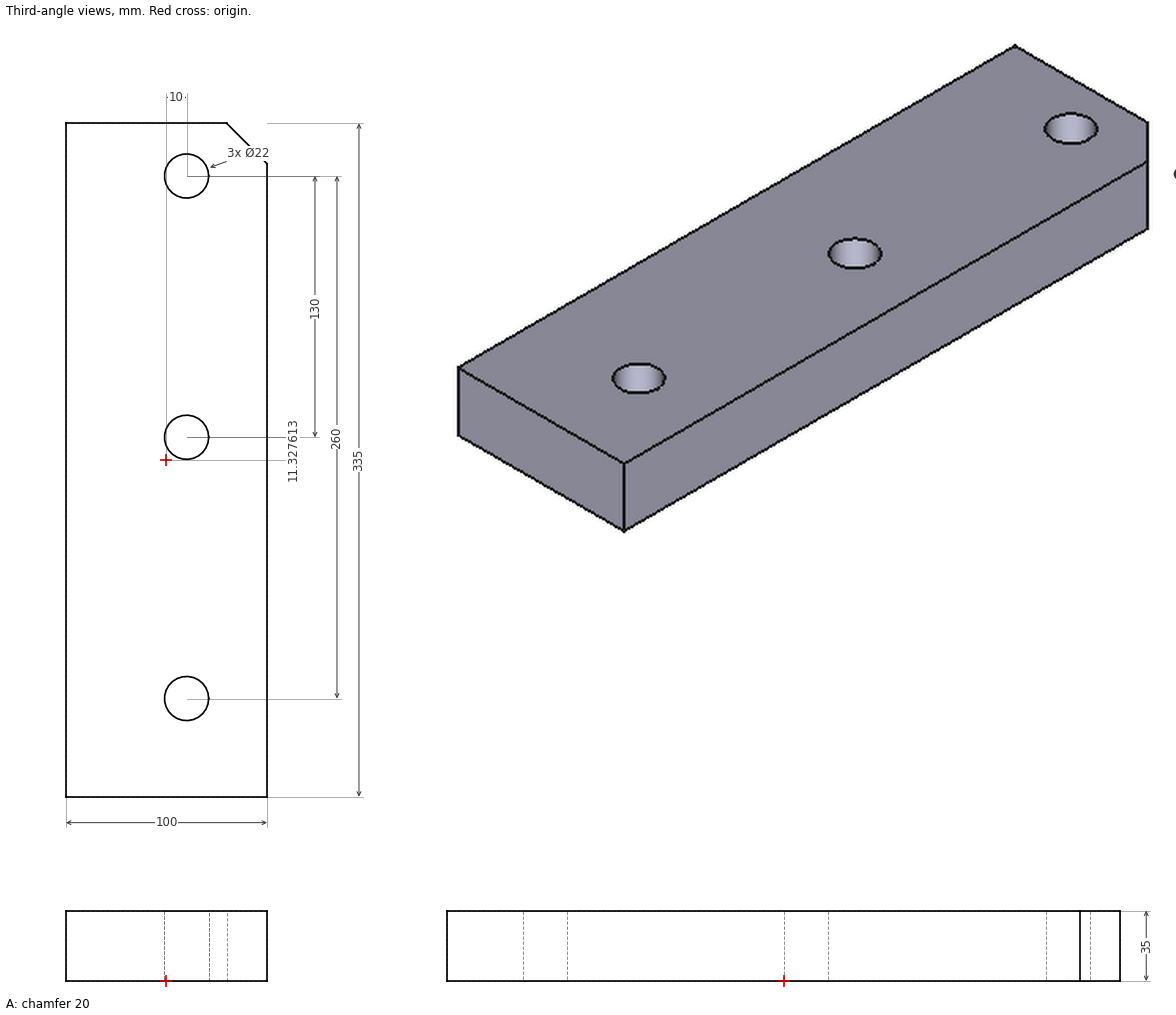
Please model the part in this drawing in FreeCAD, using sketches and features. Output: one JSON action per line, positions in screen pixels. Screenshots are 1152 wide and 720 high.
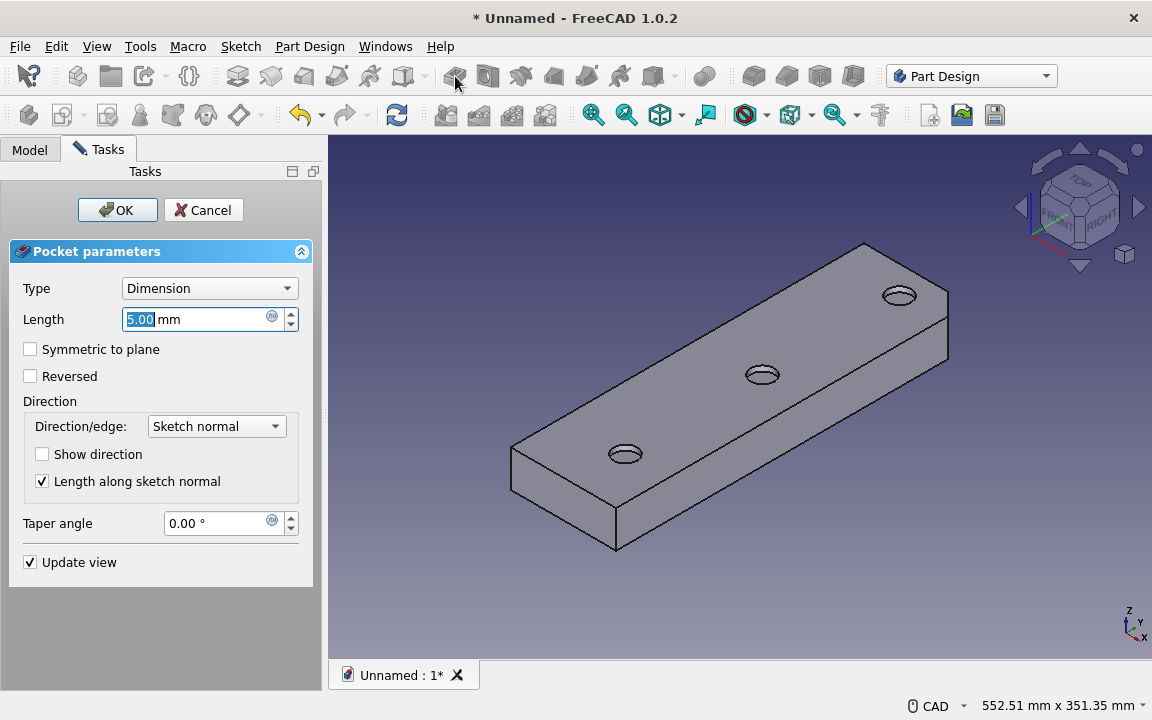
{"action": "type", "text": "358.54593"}
{"action": "key", "text": "Tab"}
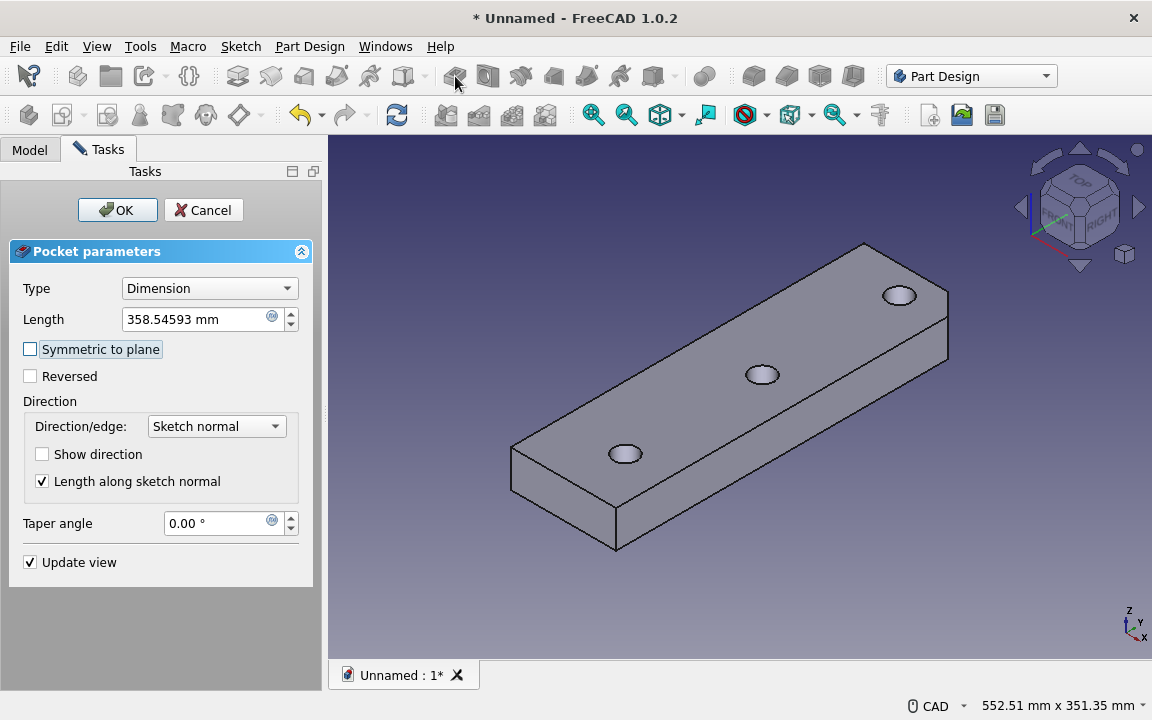
{"action": "left_click", "coordinate": [31, 349]}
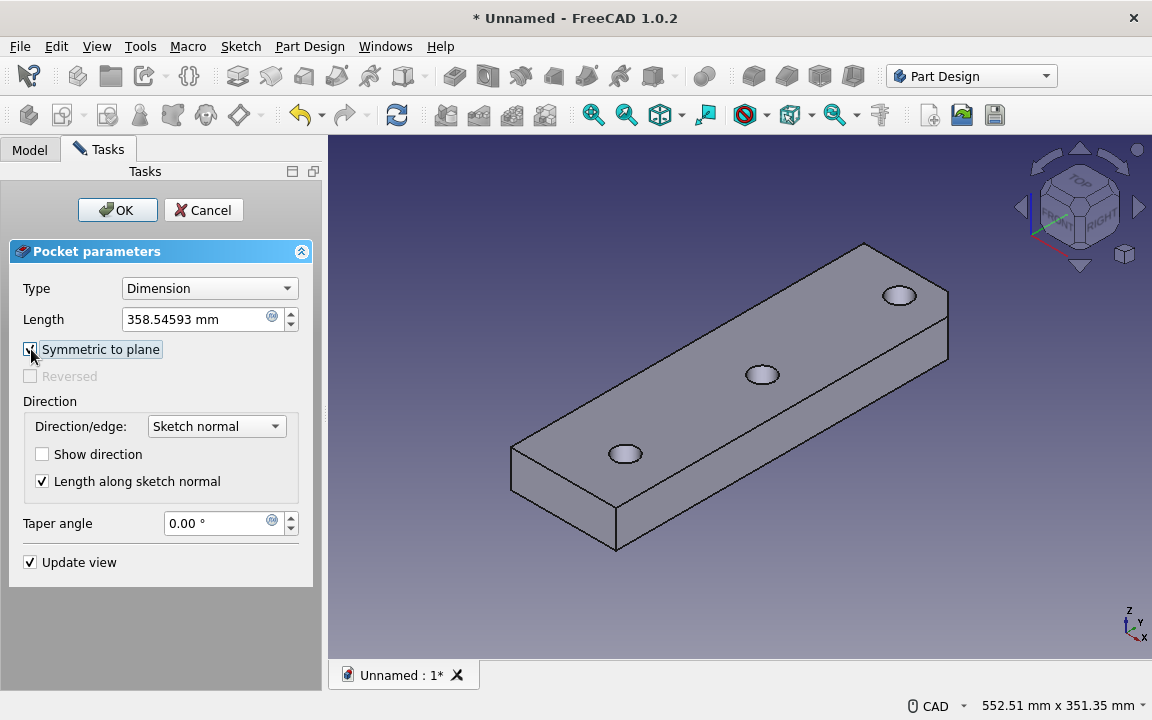
{"action": "left_click", "coordinate": [118, 210]}